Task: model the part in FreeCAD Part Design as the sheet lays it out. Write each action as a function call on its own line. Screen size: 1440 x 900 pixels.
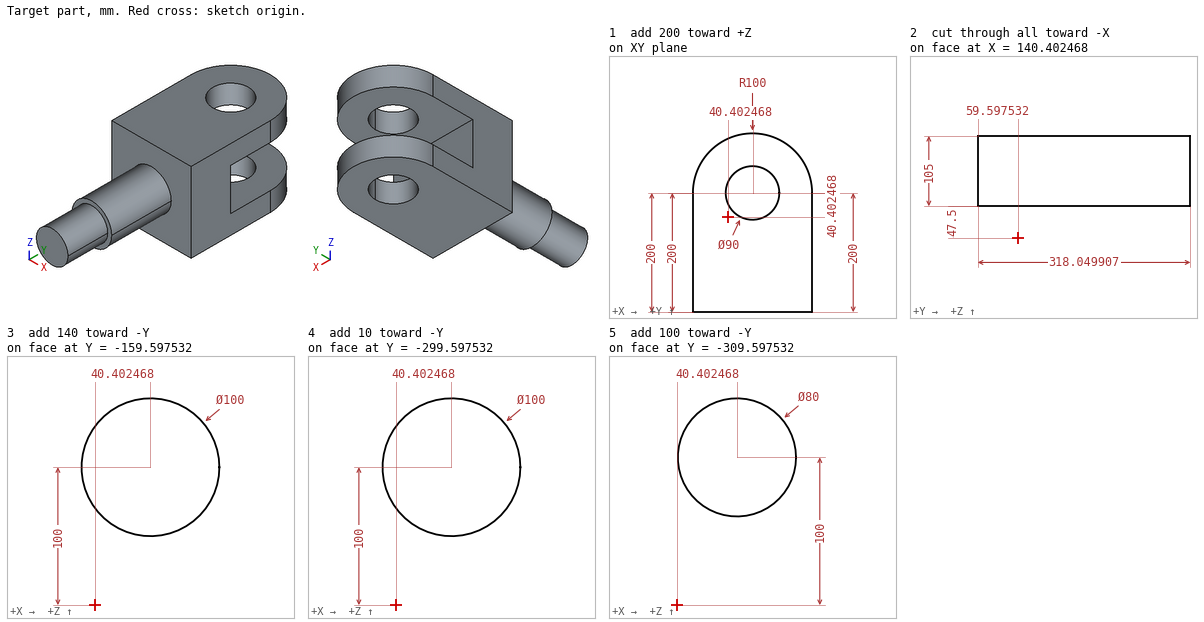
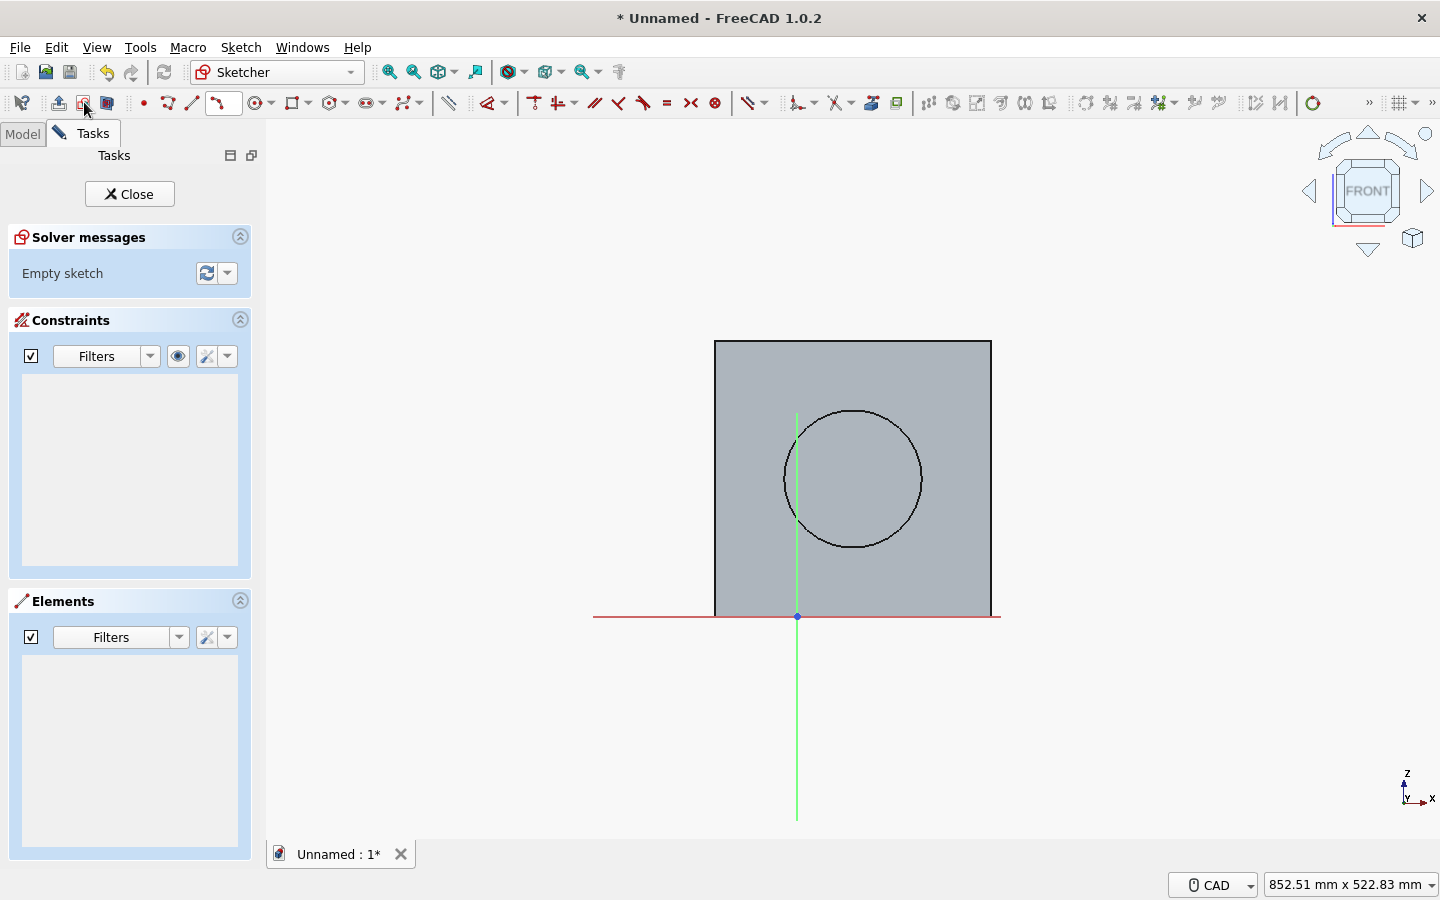
scroll(909, 542, up, 4)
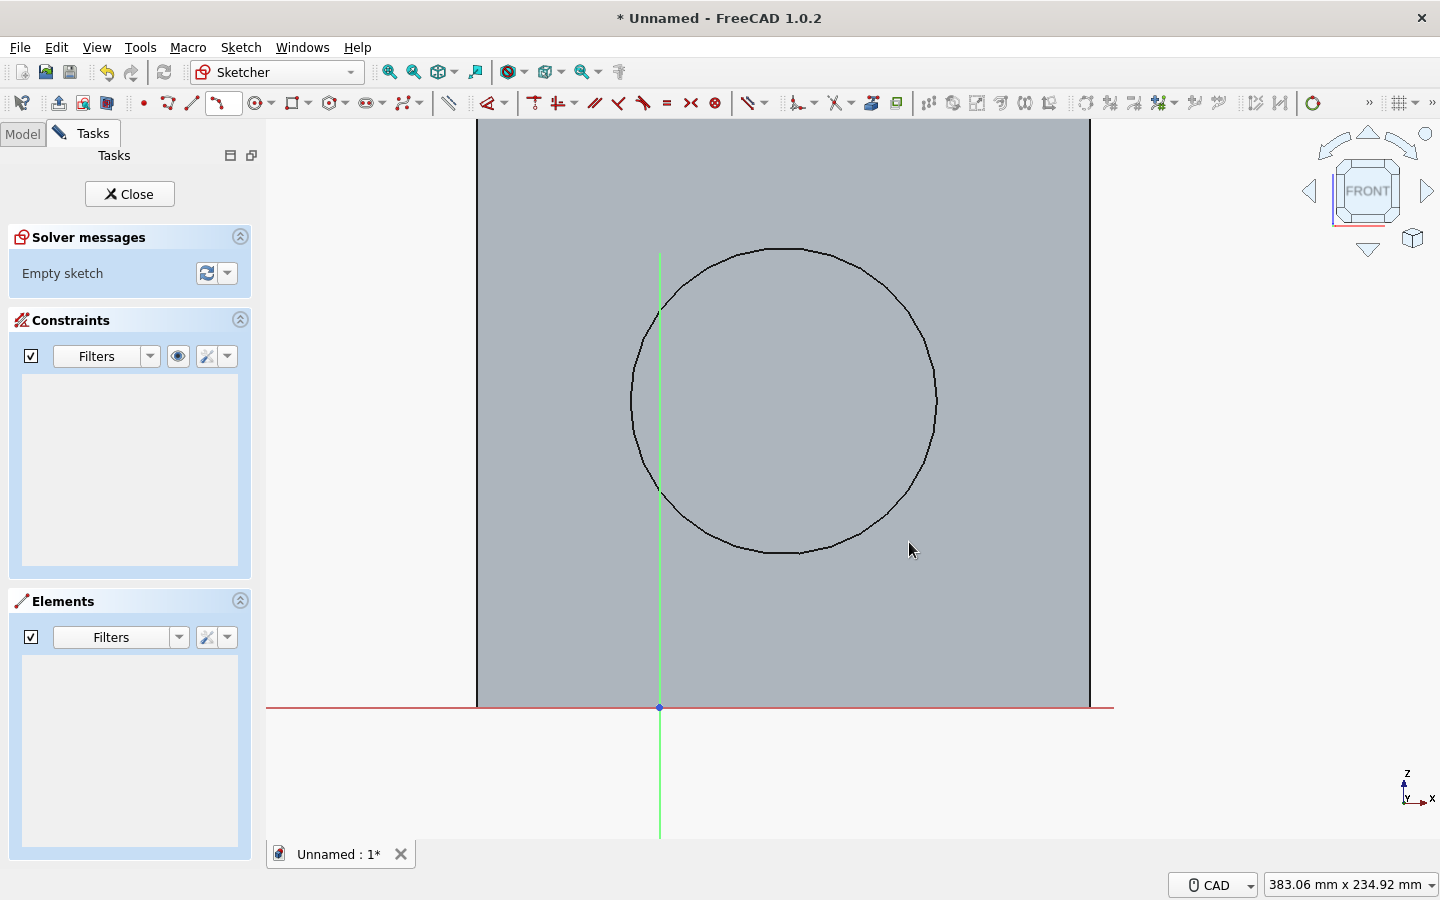
key(g)
key(c)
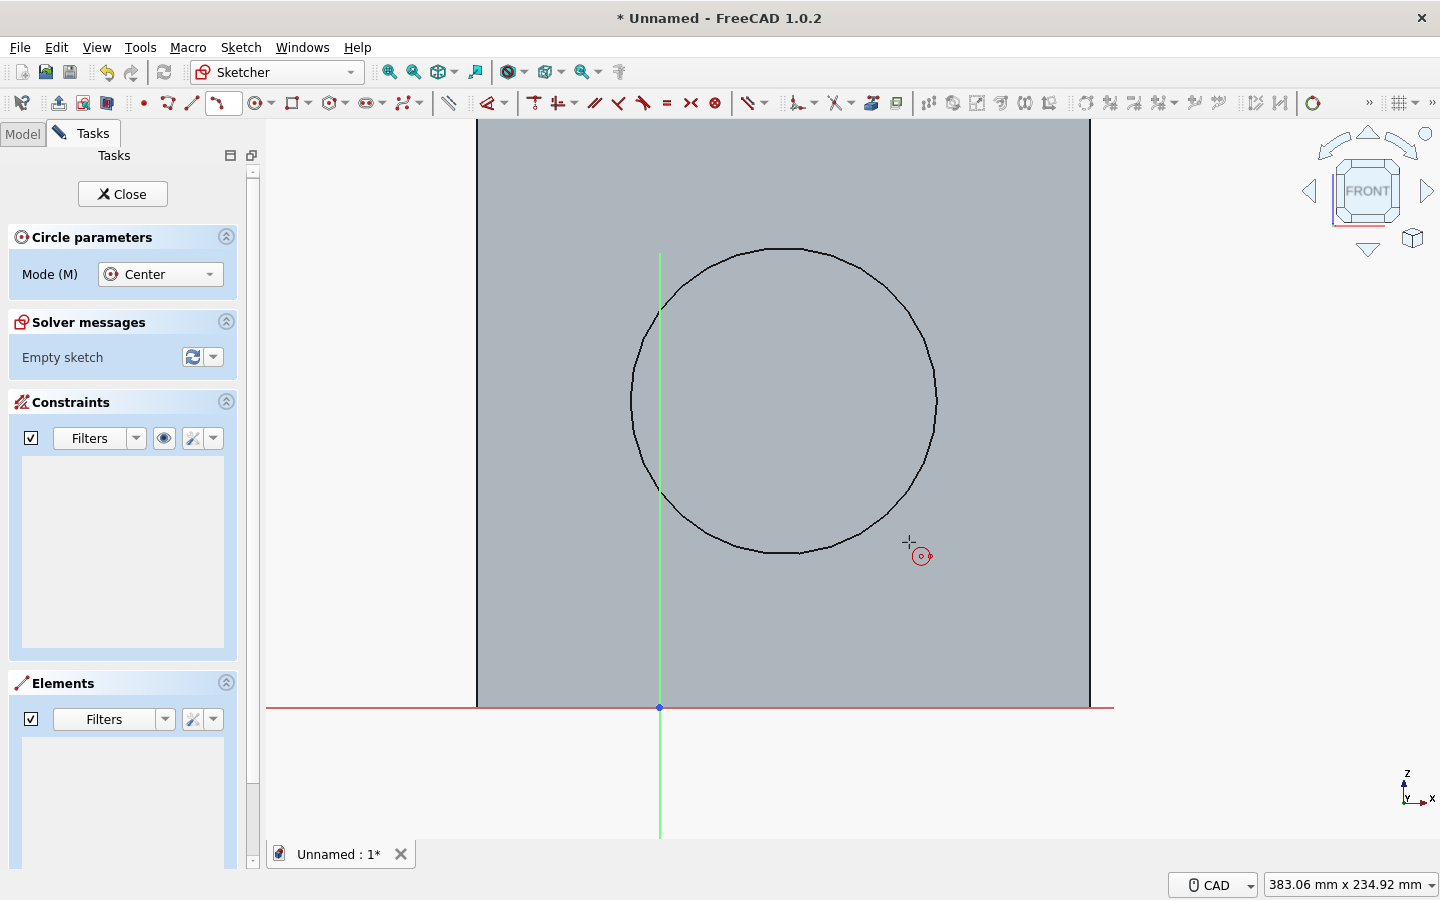
click(784, 401)
click(892, 293)
key(Escape)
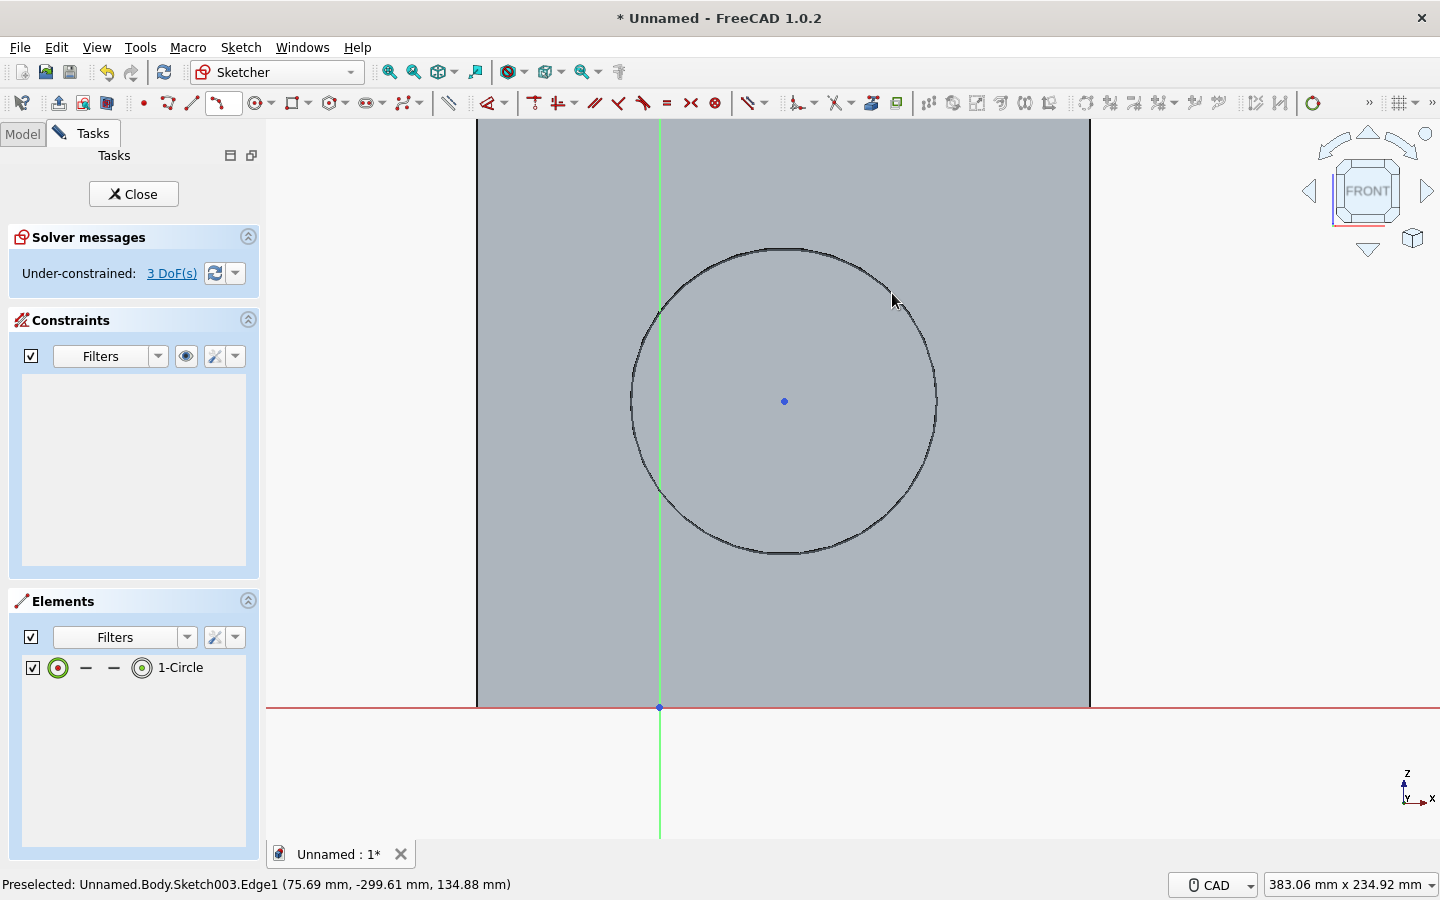
key(d)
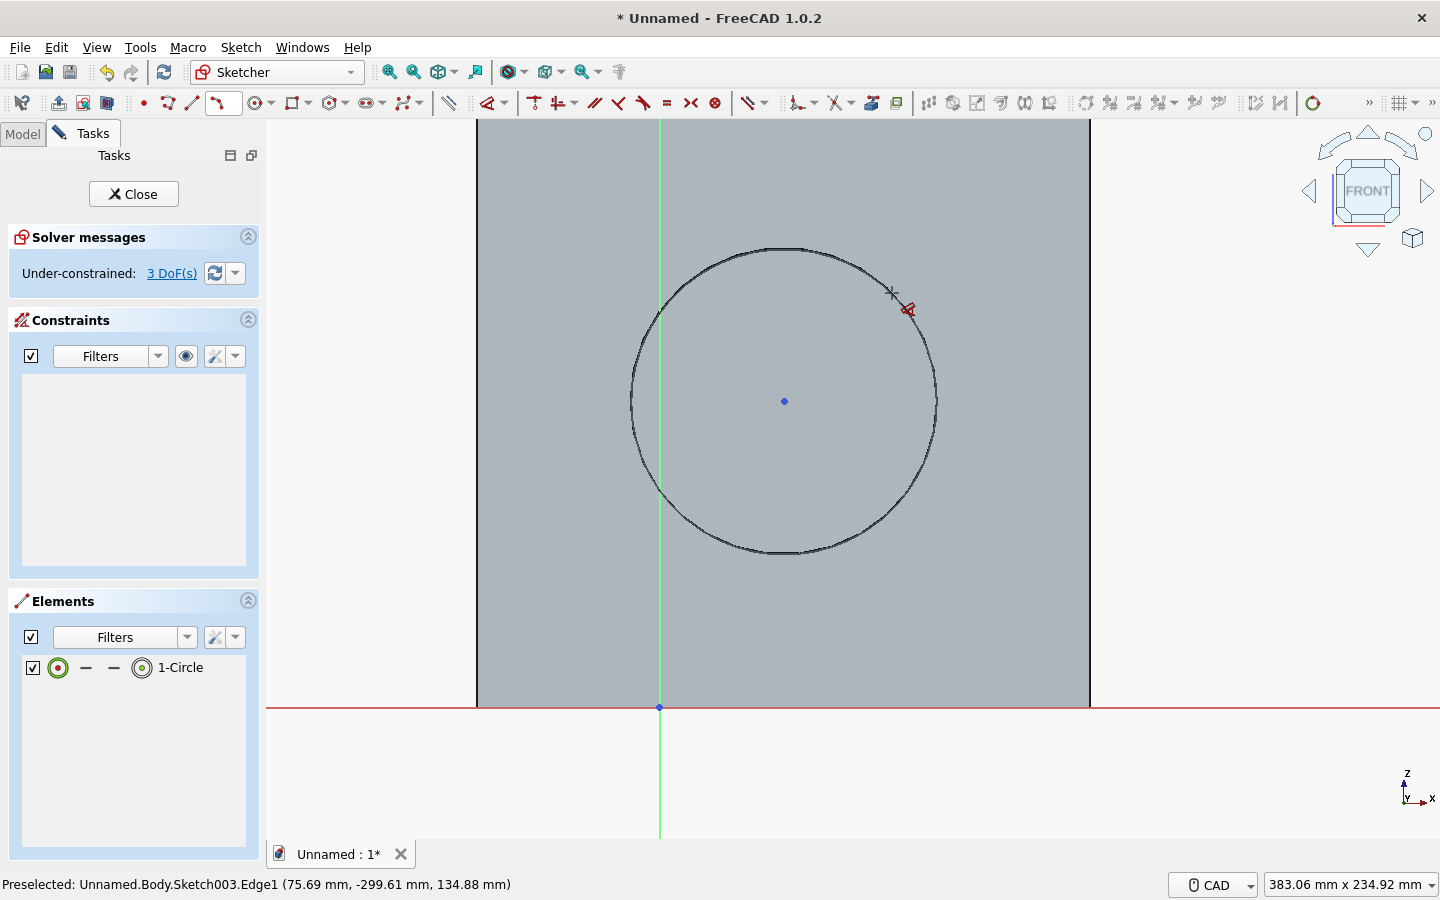
click(892, 294)
click(915, 271)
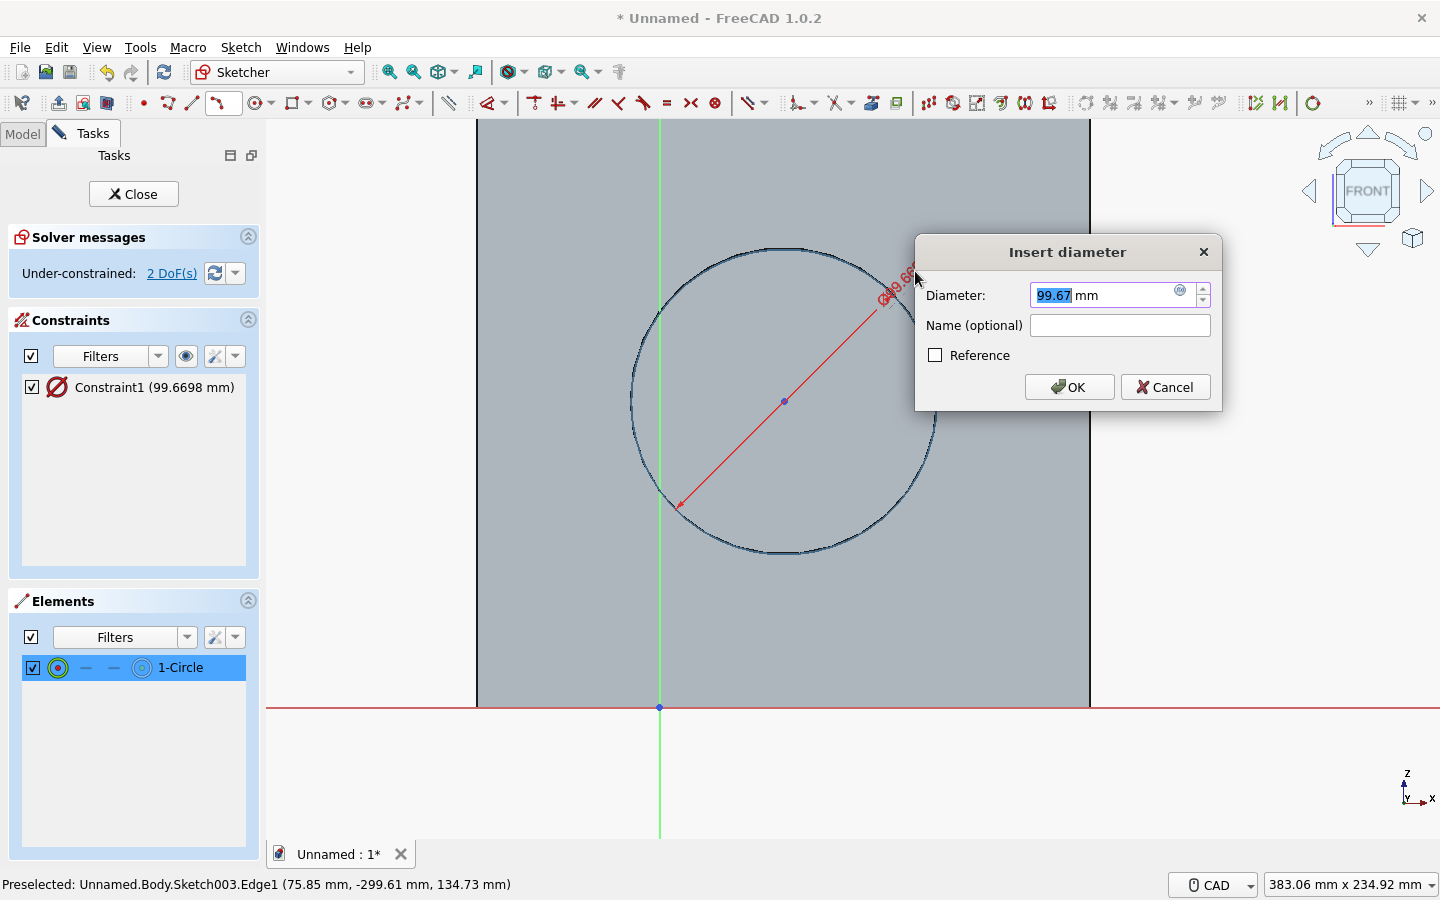
text(100)
key(Return)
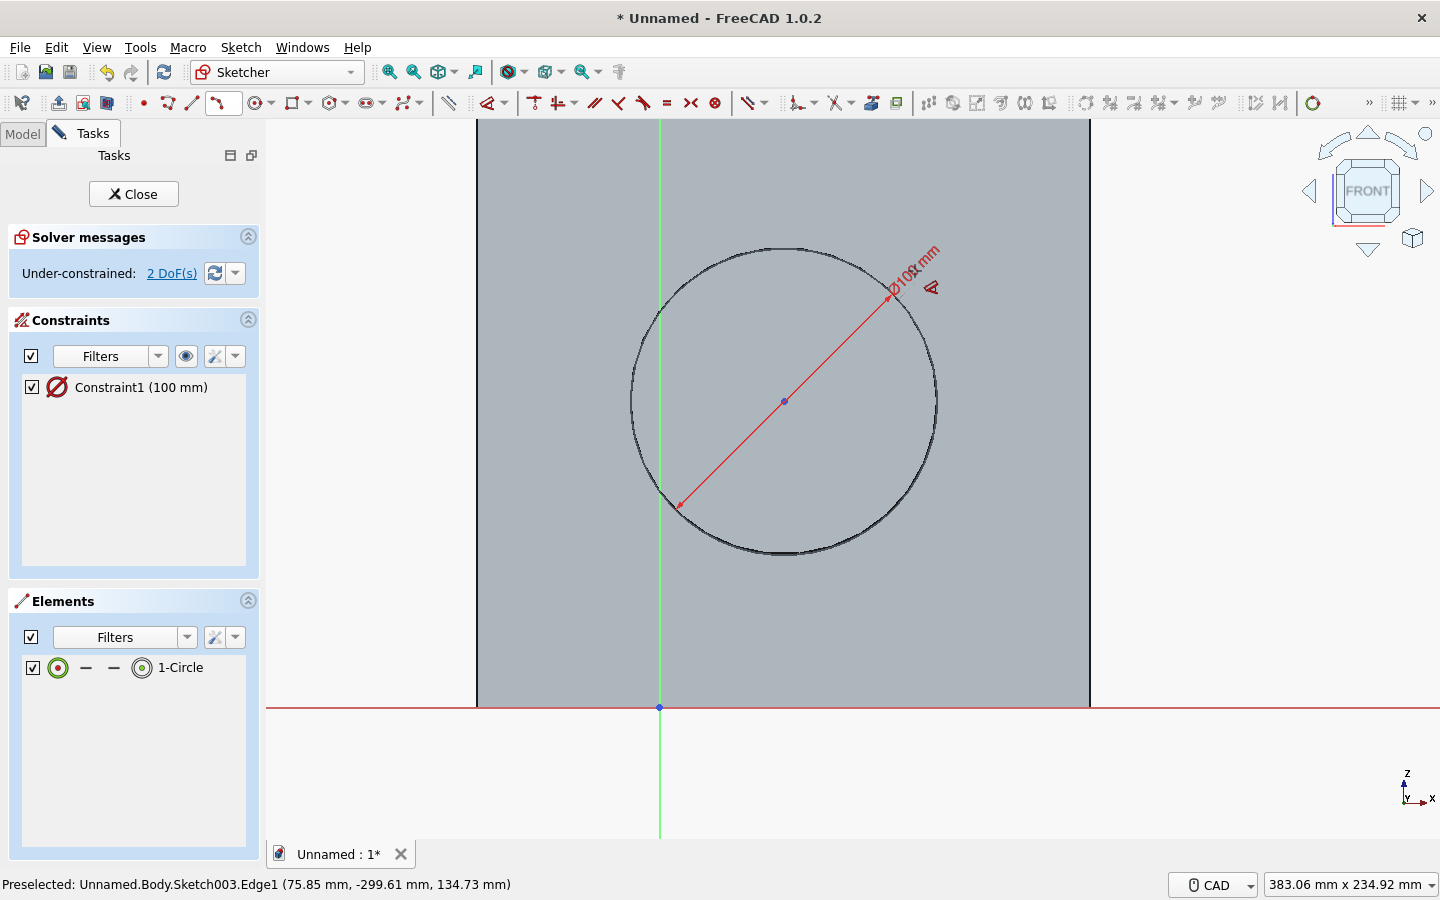
click(784, 402)
click(626, 555)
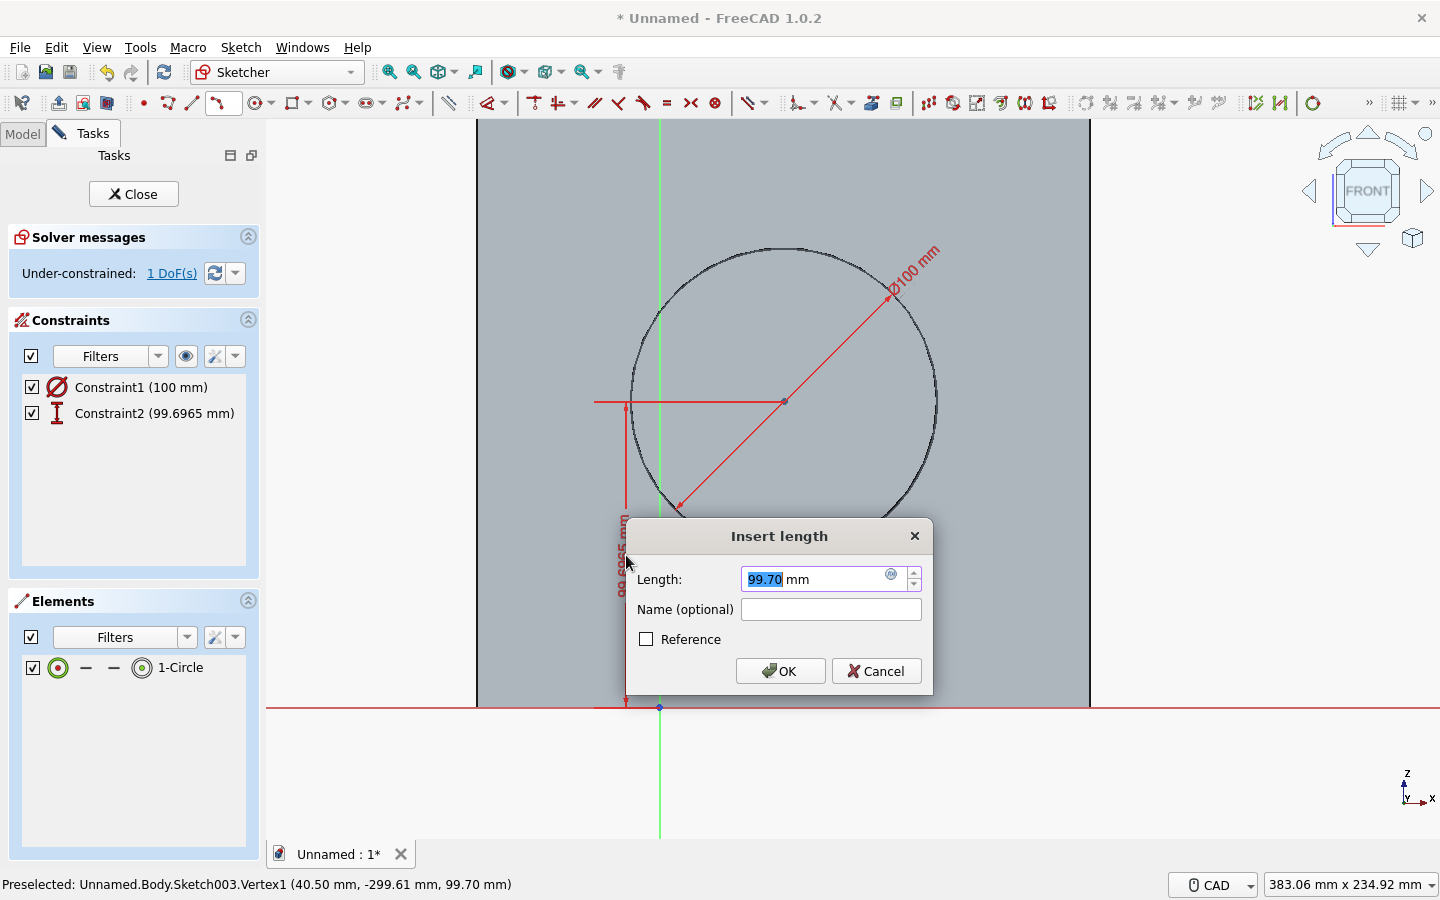
text(100)
key(Return)